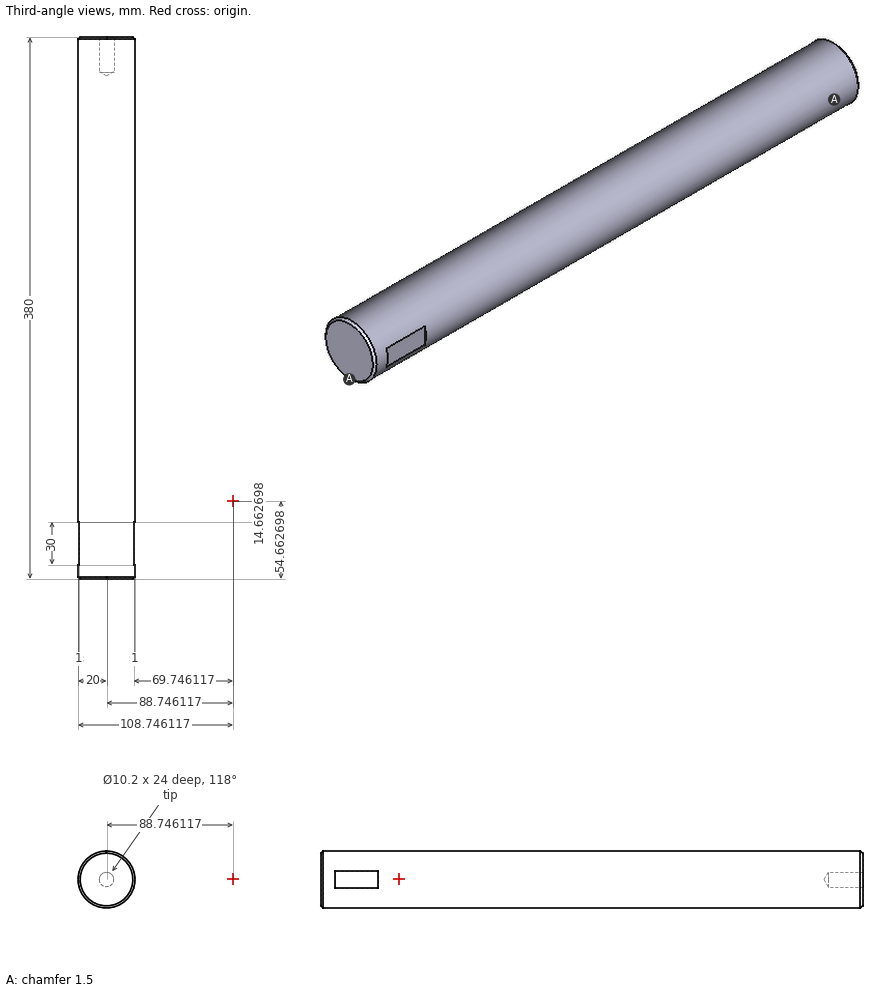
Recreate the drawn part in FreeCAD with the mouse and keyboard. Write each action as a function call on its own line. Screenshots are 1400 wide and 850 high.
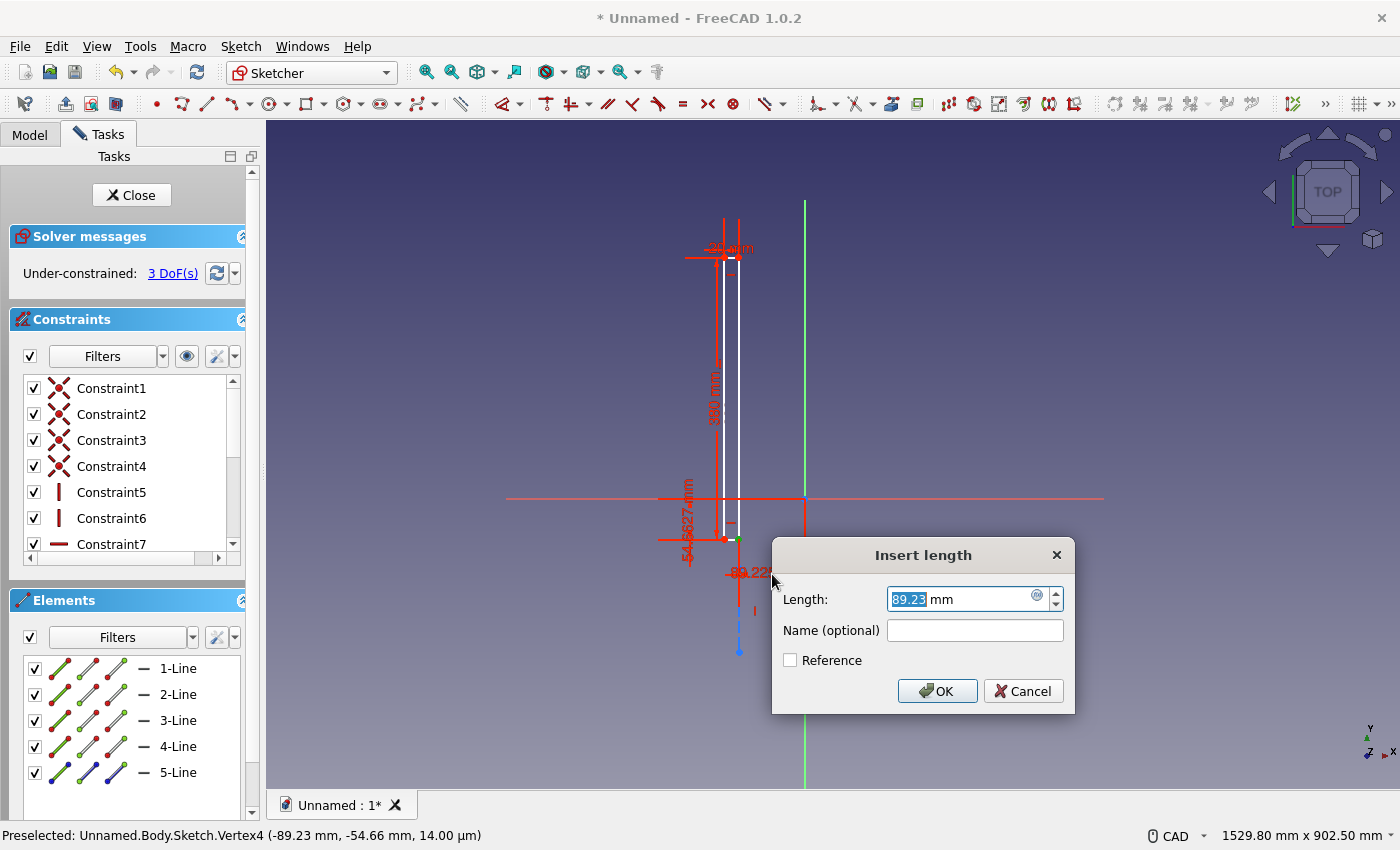
text(88.746117)
key(Return)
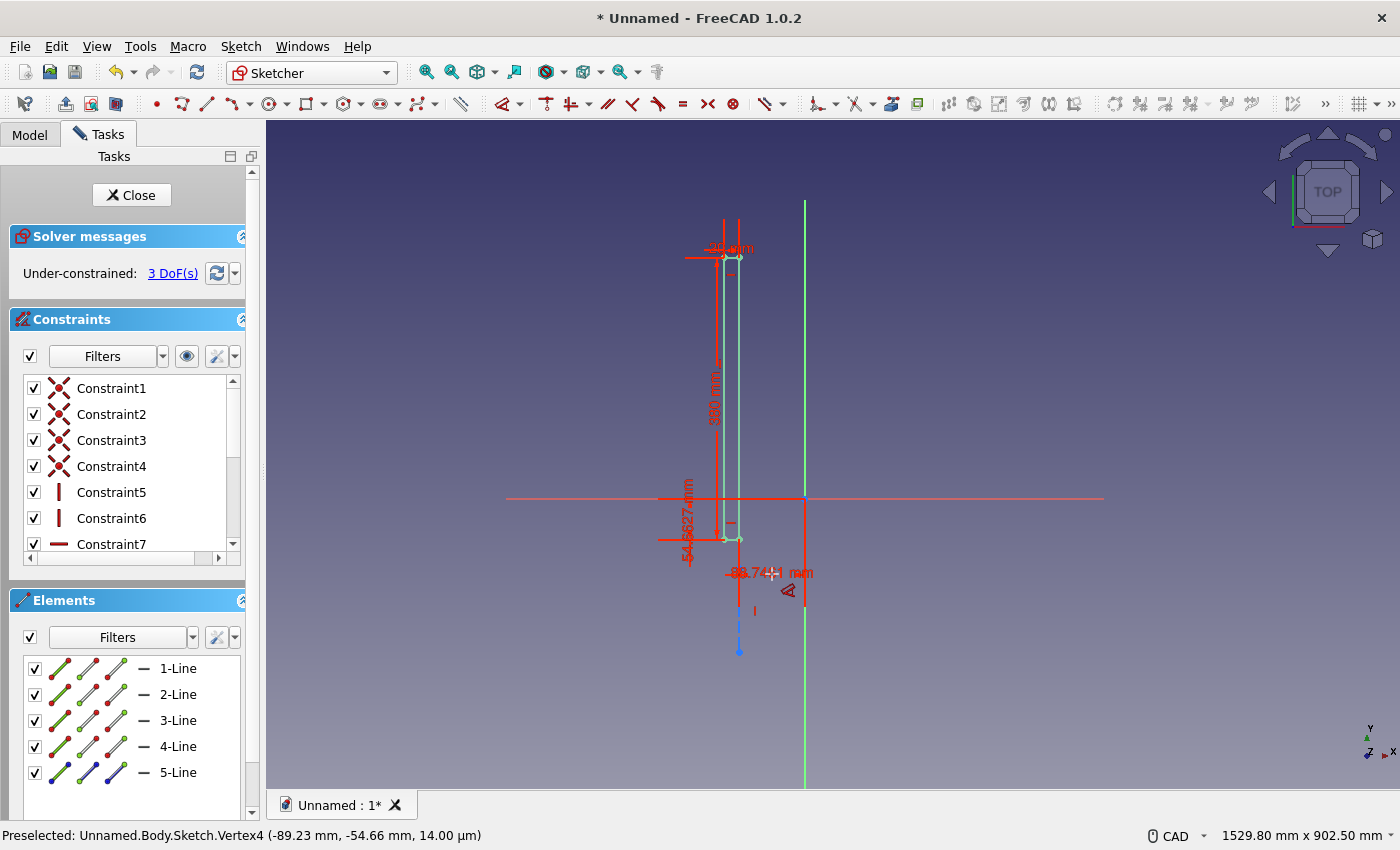
click(739, 569)
click(772, 603)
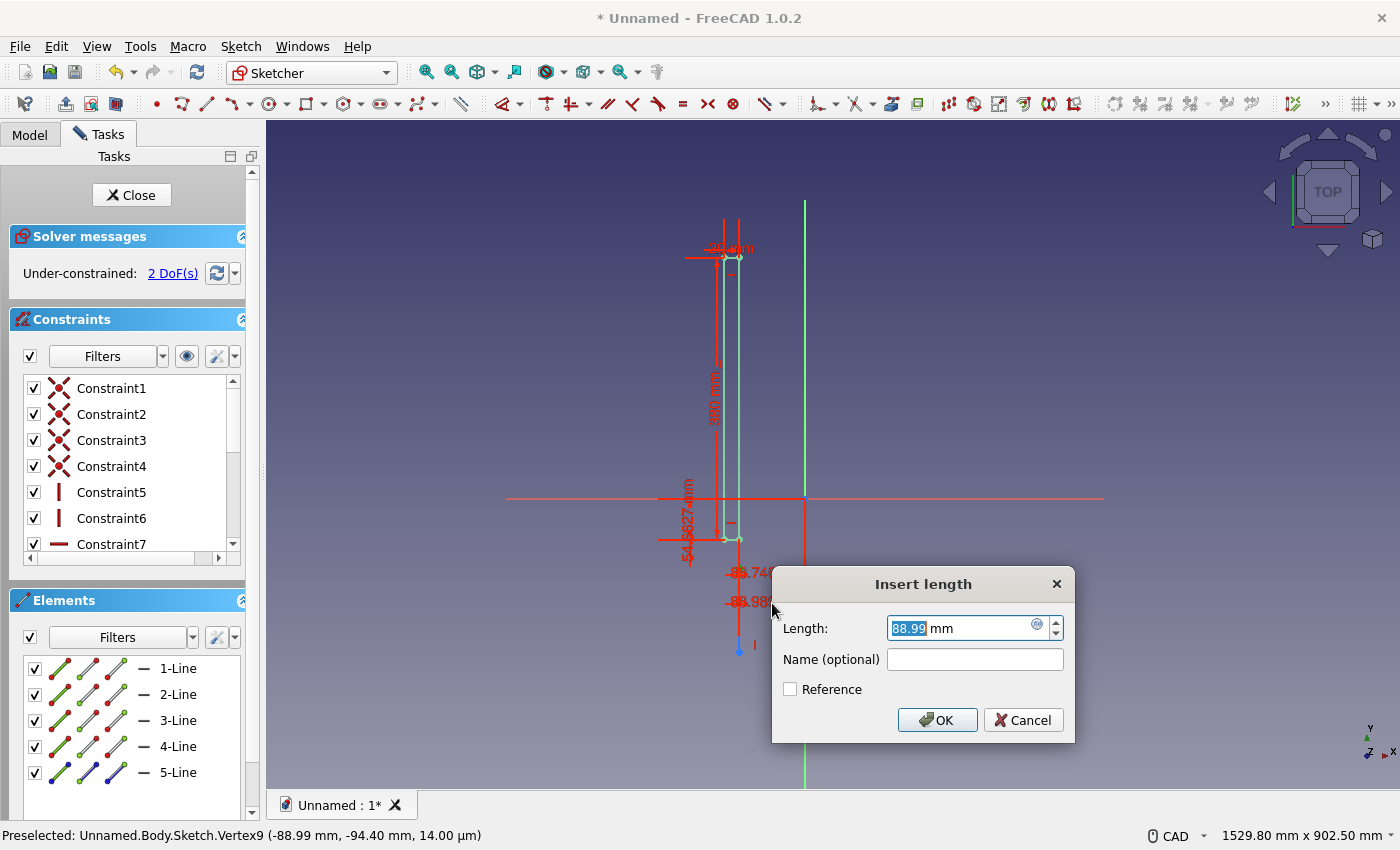
text(88.746117)
key(Return)
key(Escape)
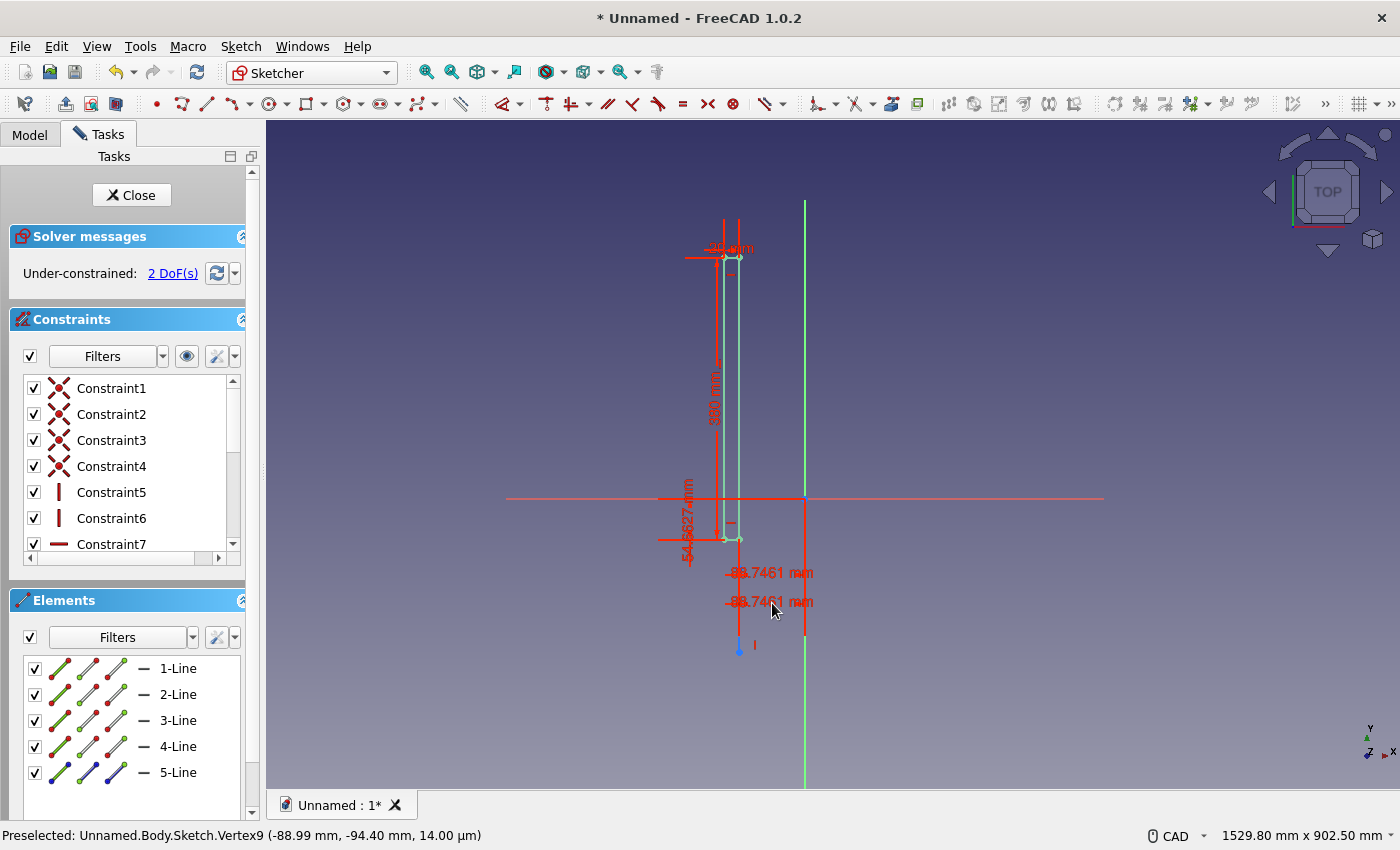
click(132, 195)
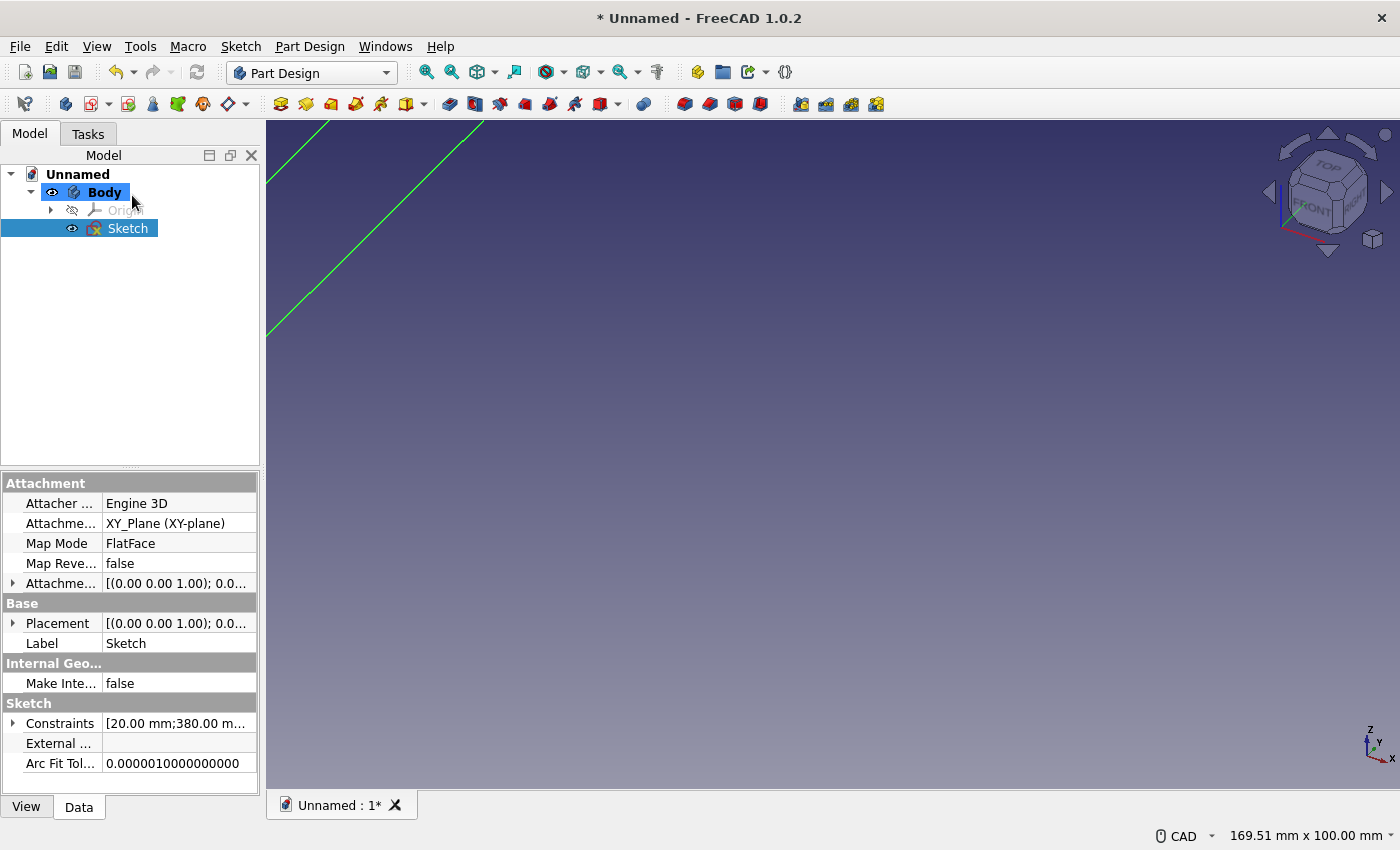
click(306, 104)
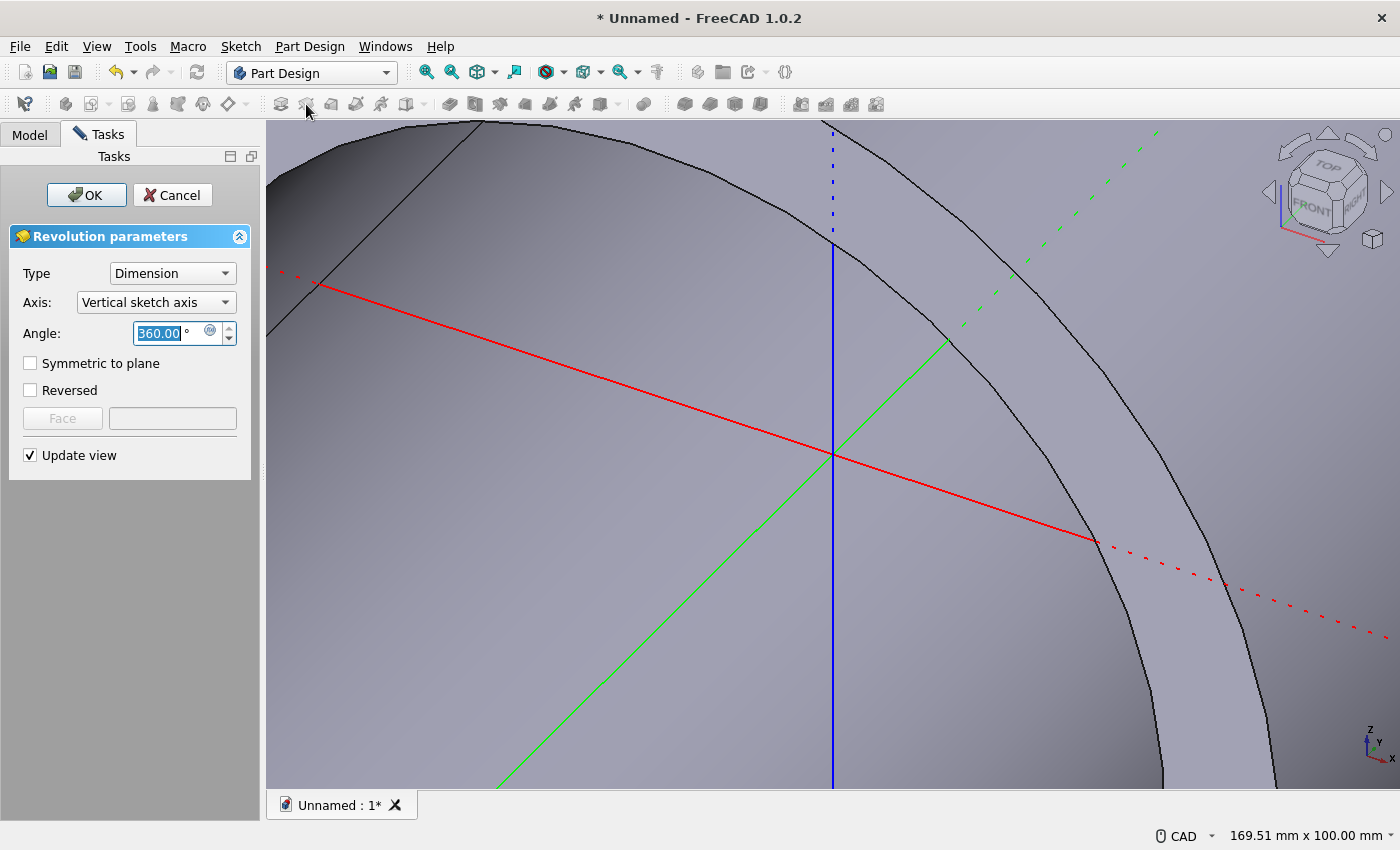
click(157, 302)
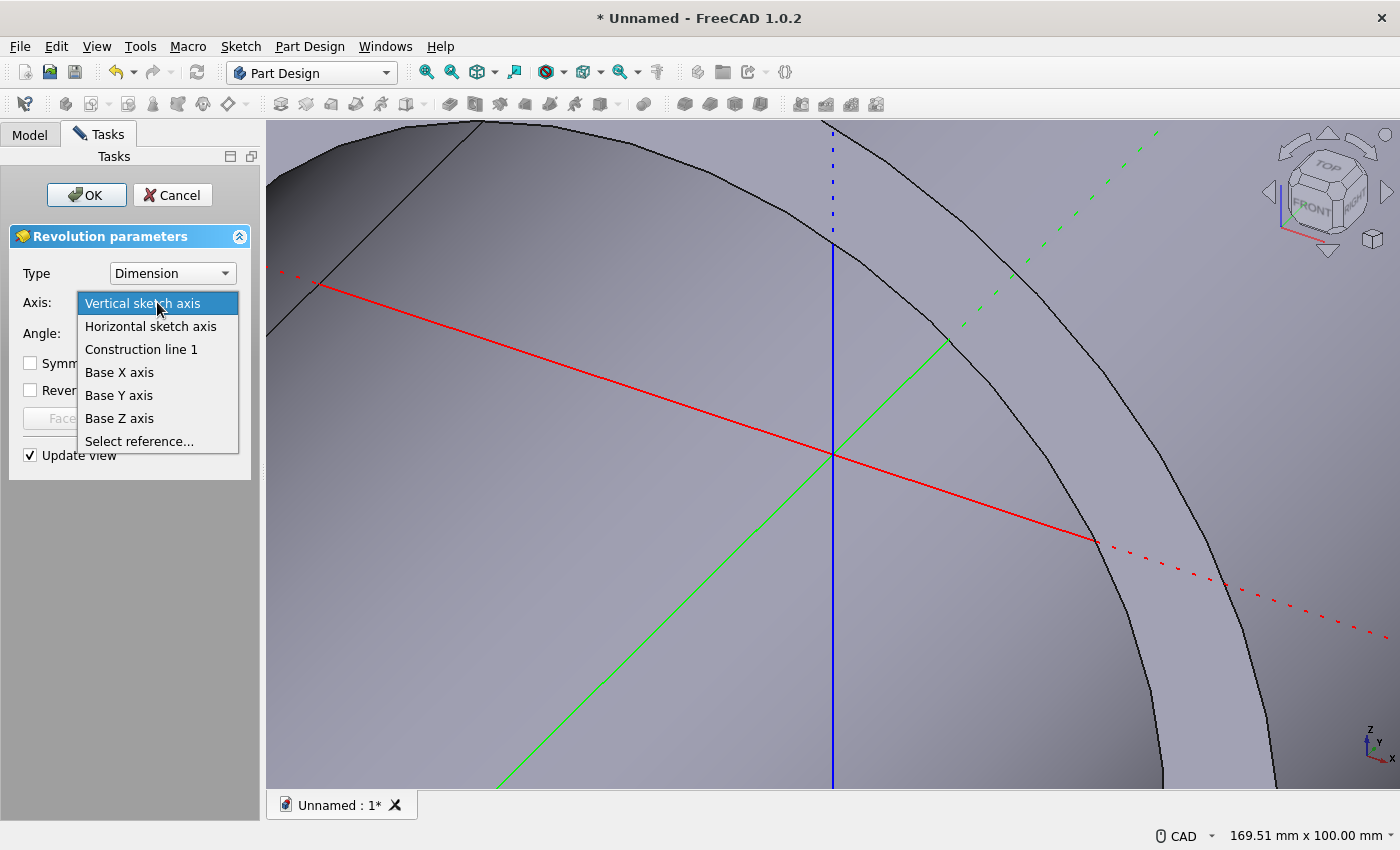
click(156, 350)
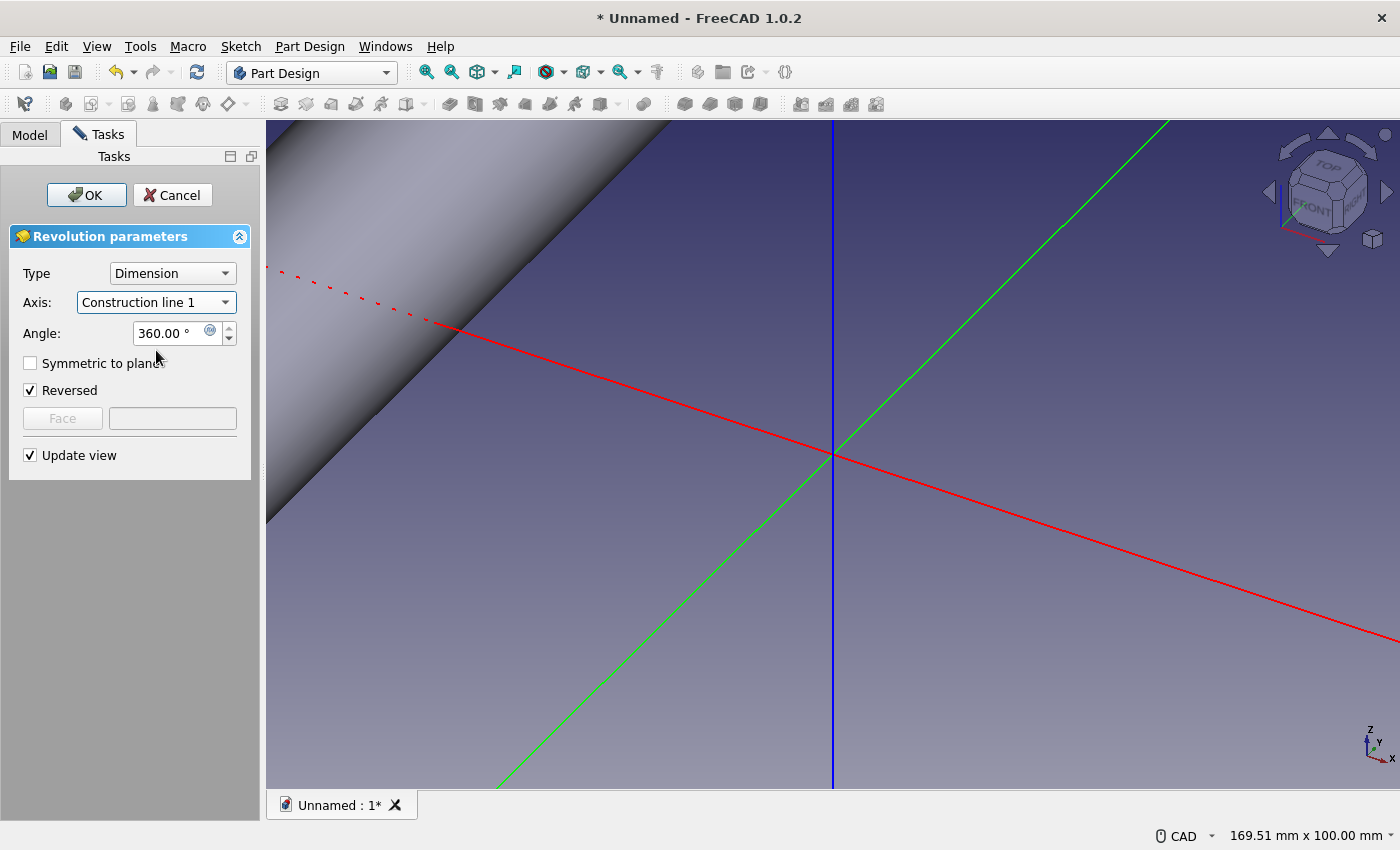
click(87, 195)